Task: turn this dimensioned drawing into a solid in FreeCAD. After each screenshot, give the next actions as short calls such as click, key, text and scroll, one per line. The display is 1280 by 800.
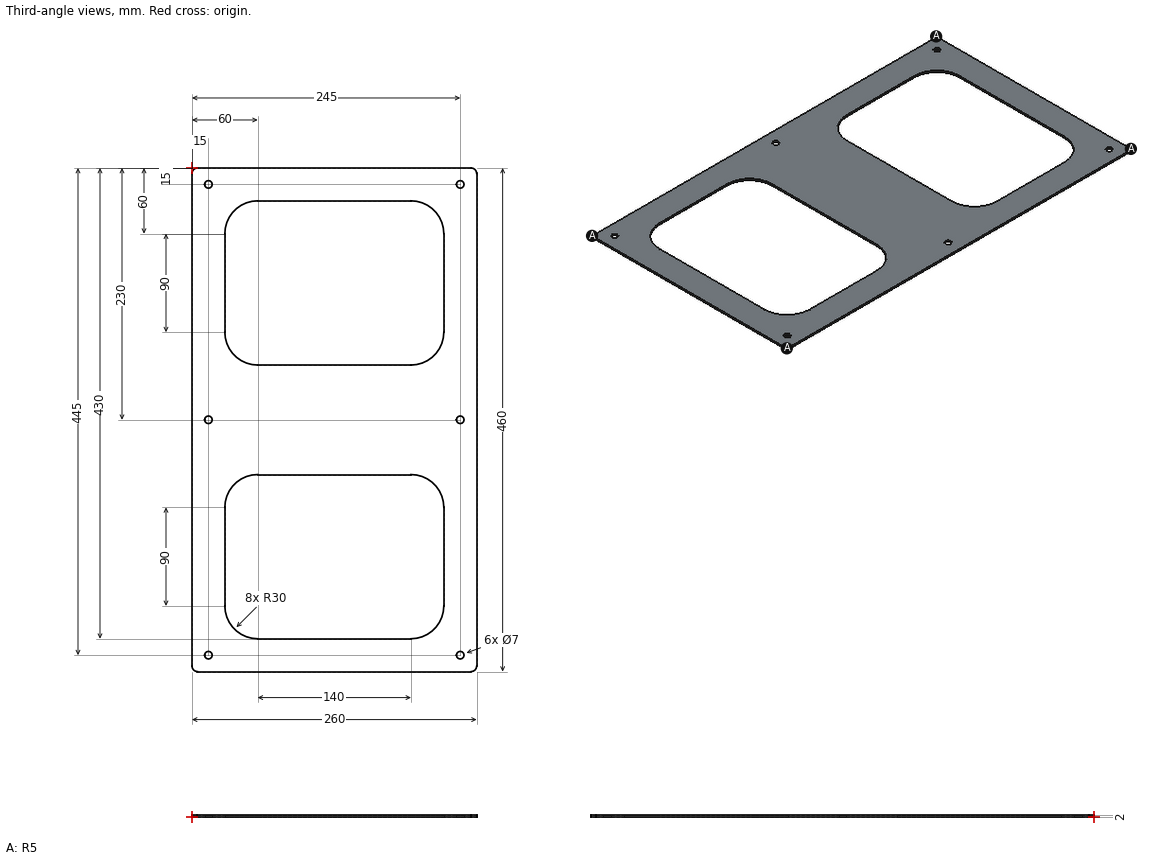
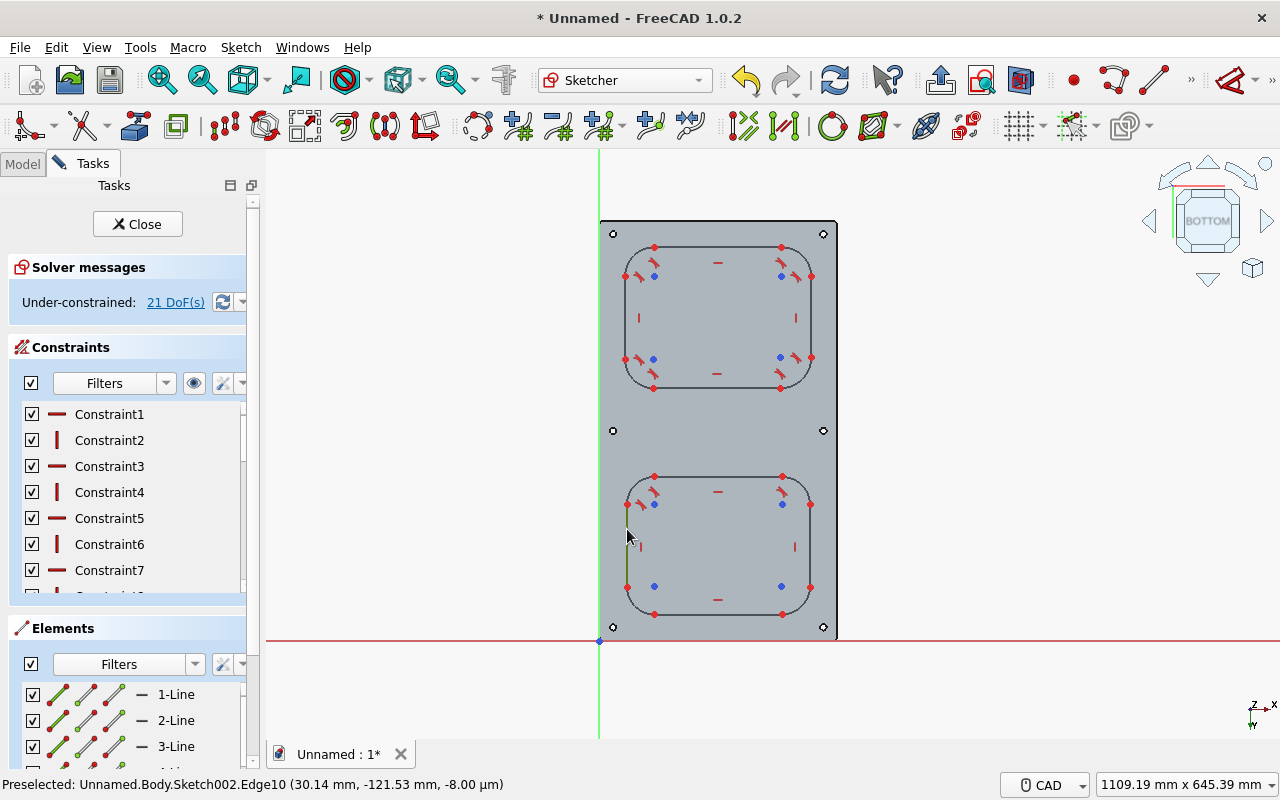
click(630, 600)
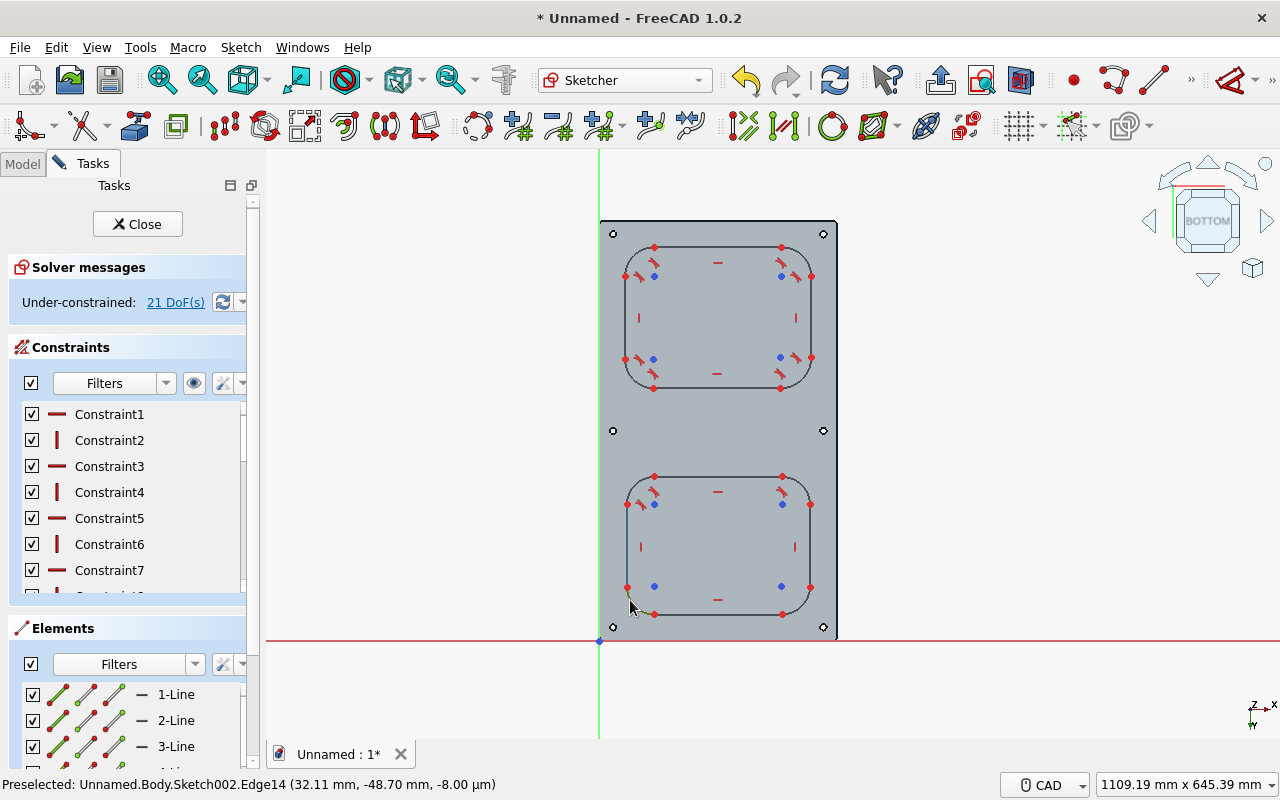
key(t)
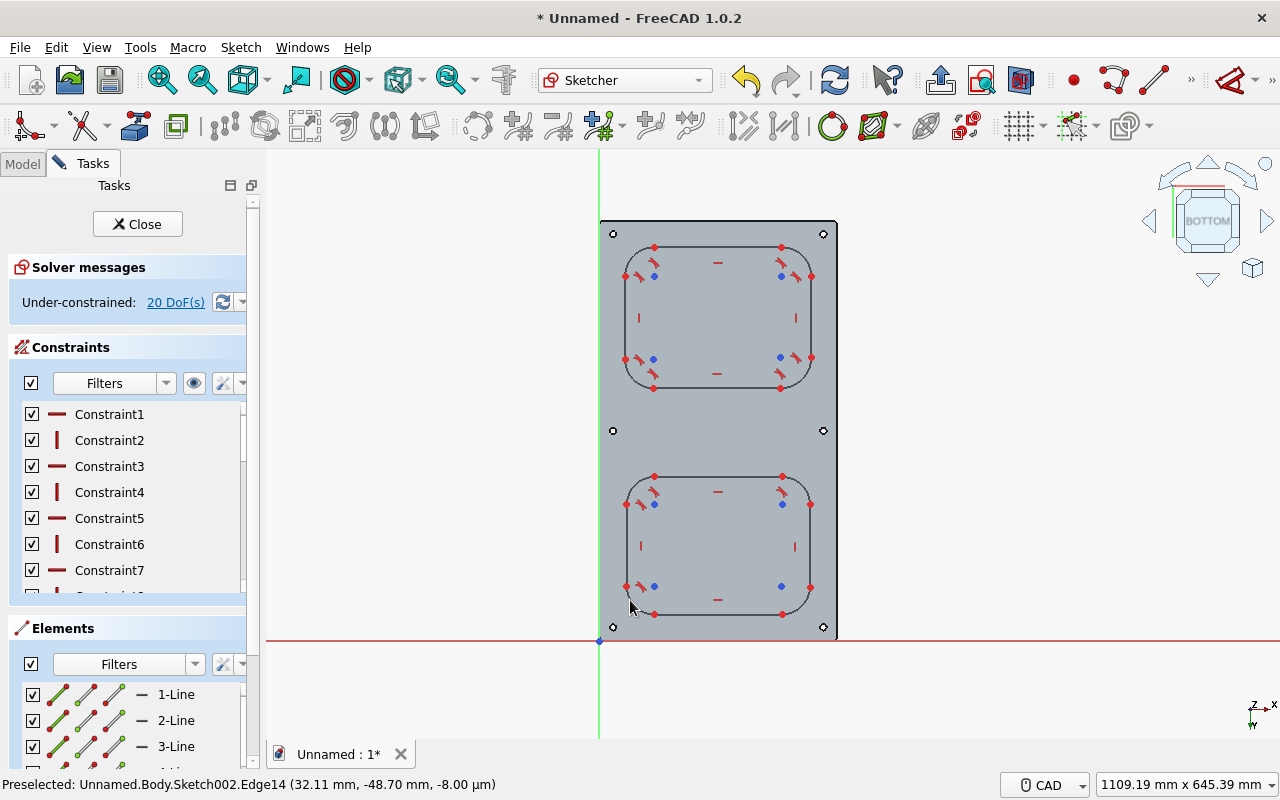
click(692, 615)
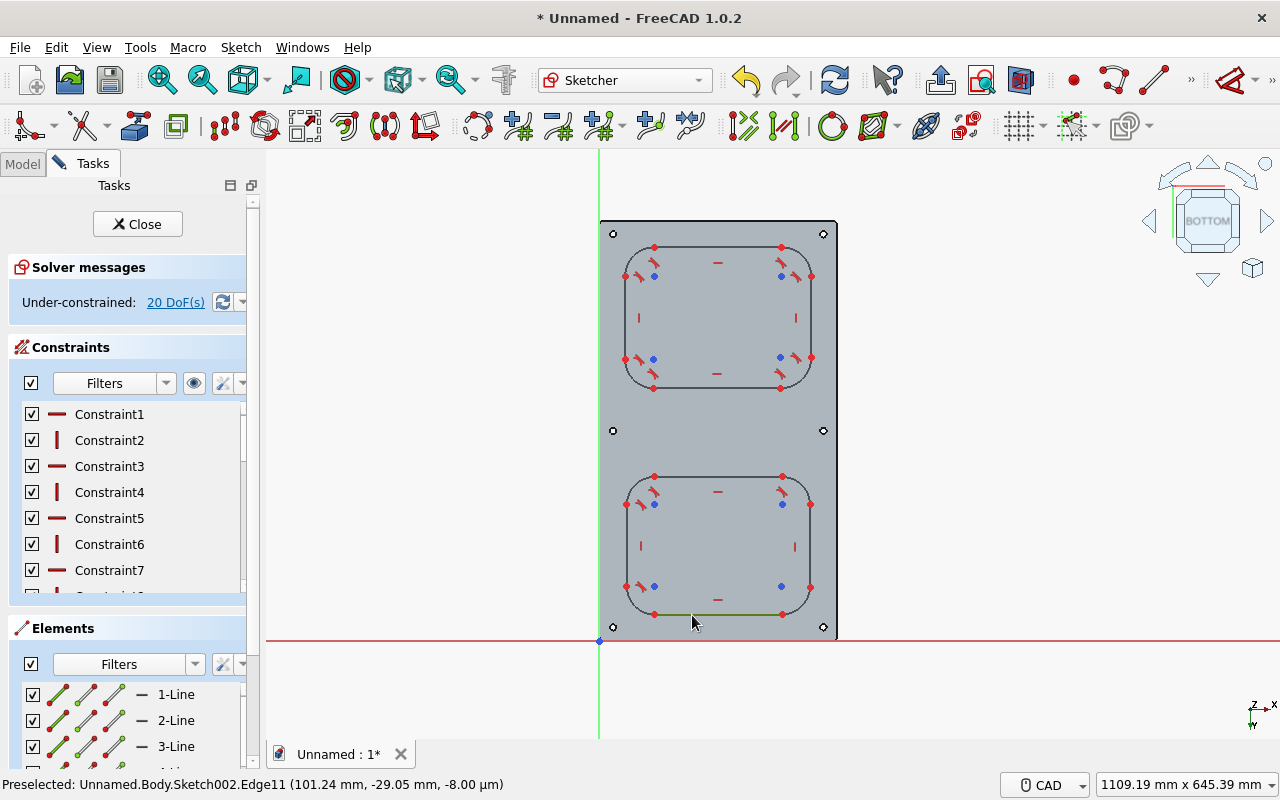
click(630, 599)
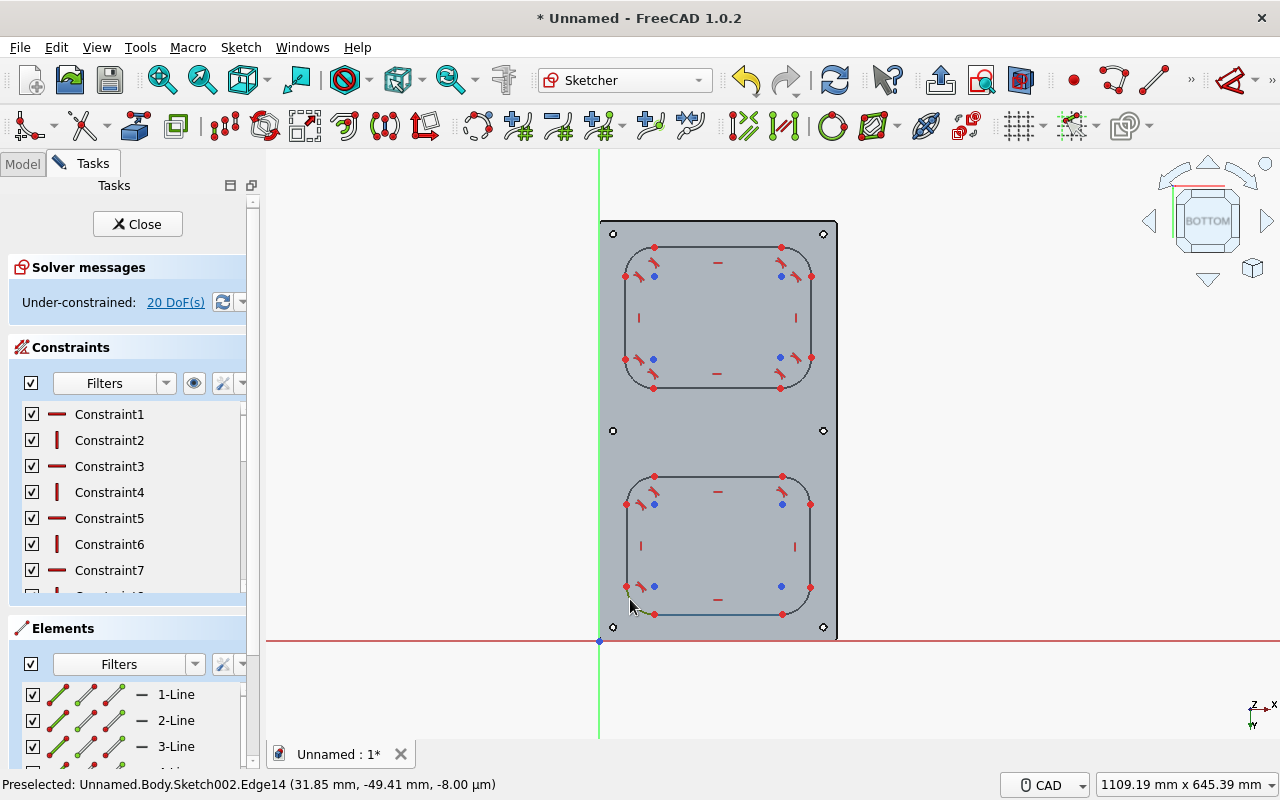
key(t)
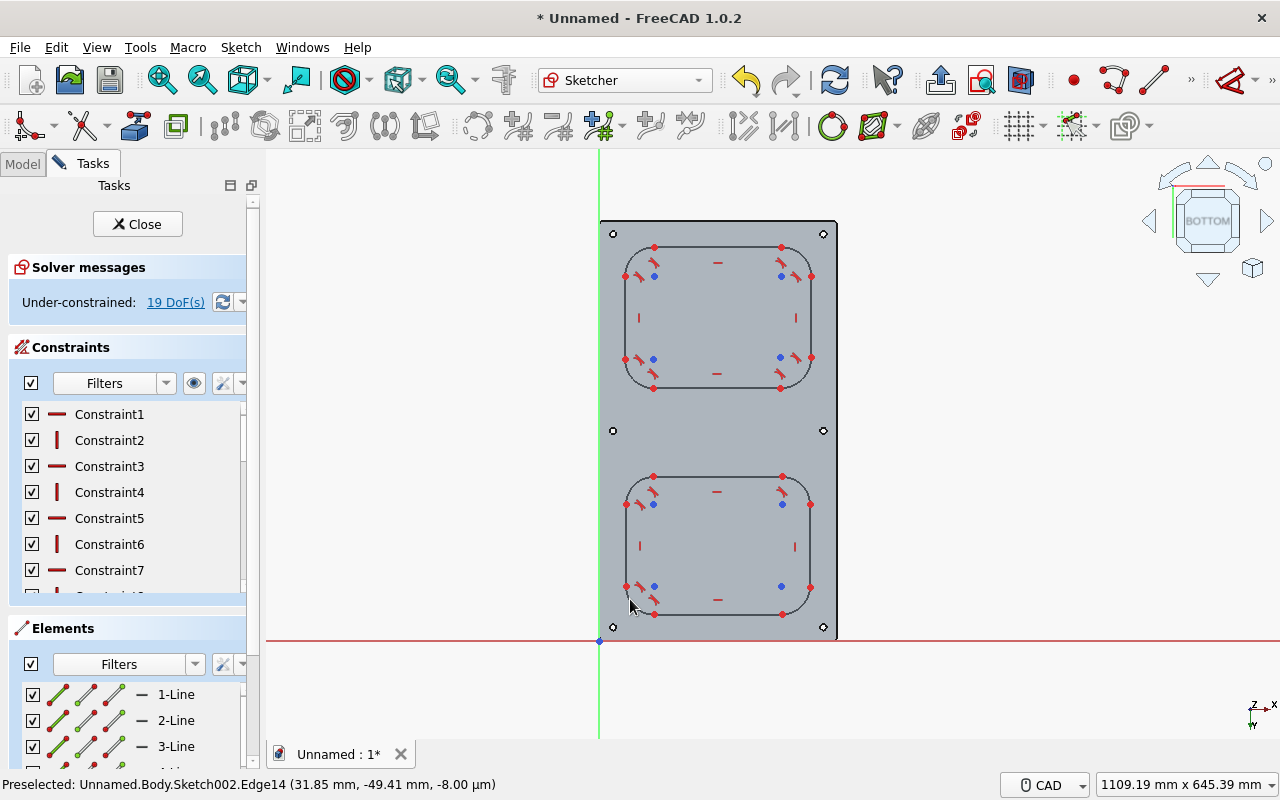
click(692, 615)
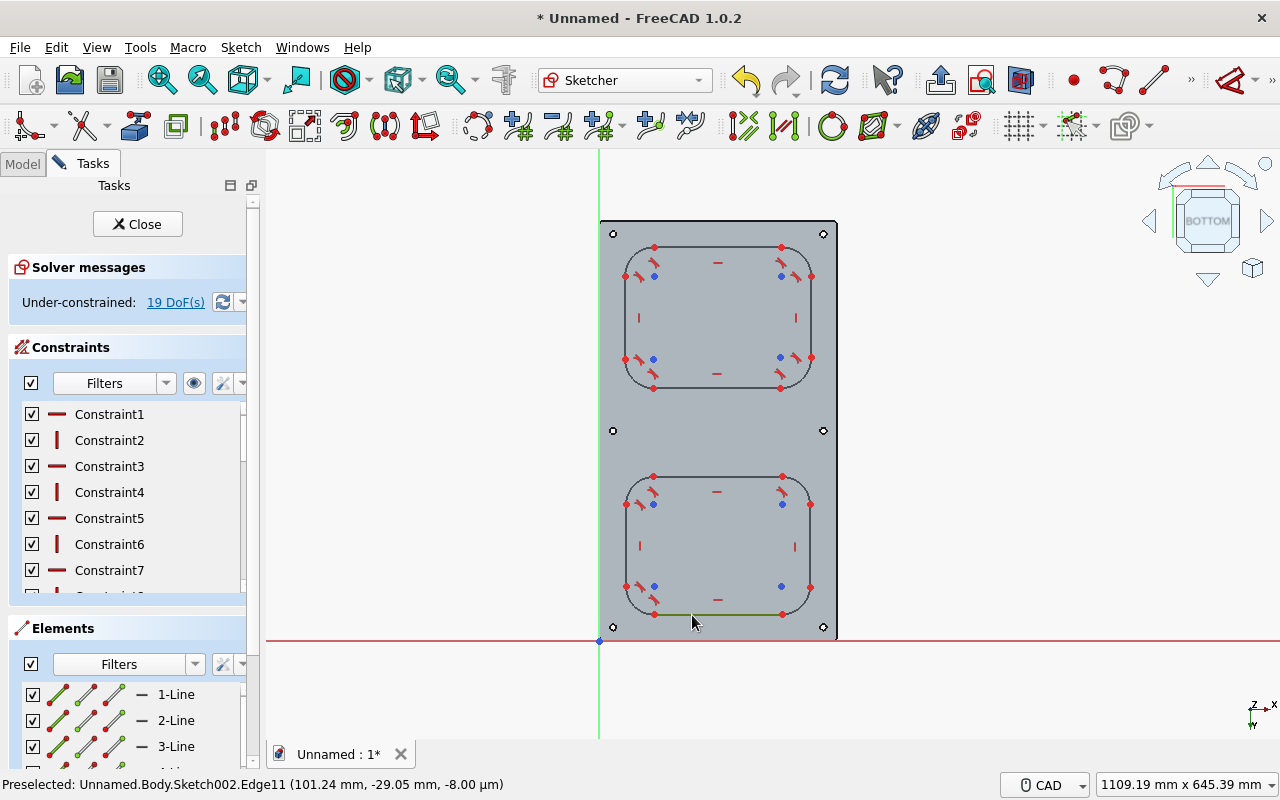
click(794, 611)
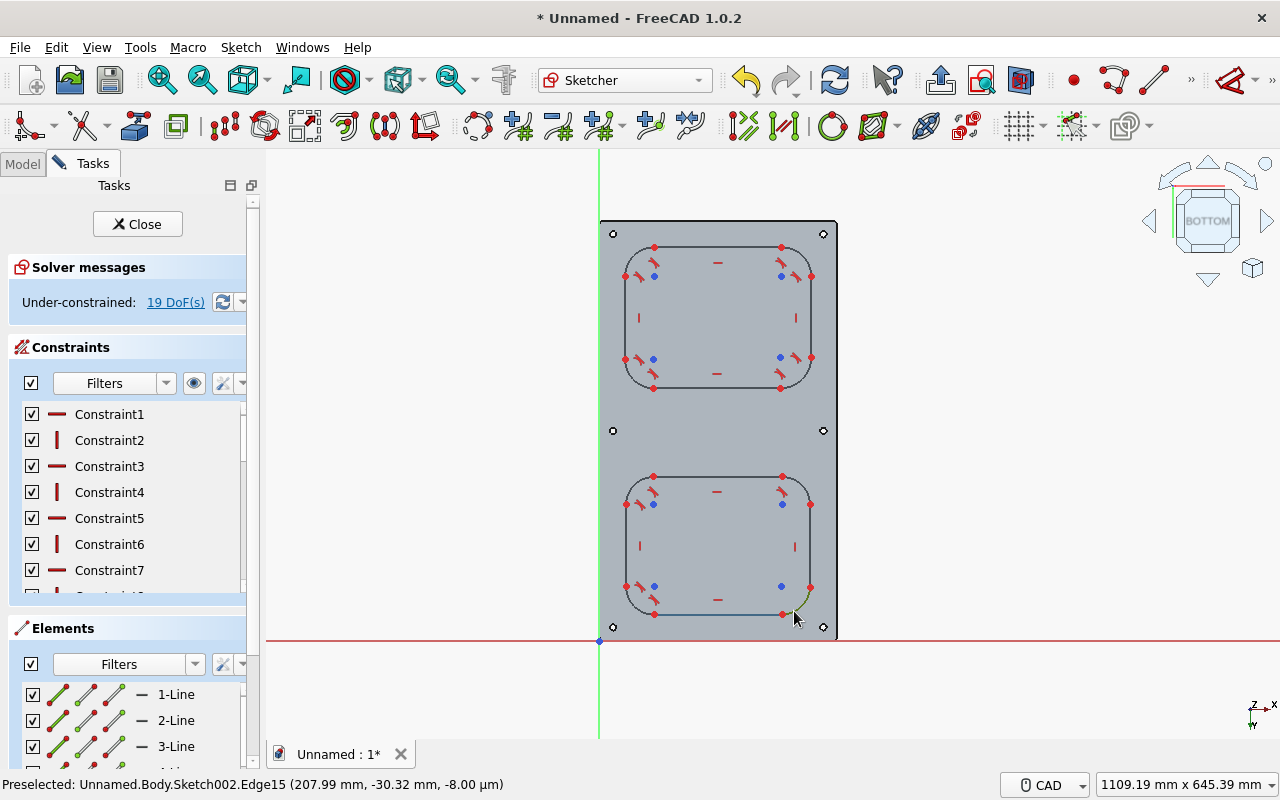
key(t)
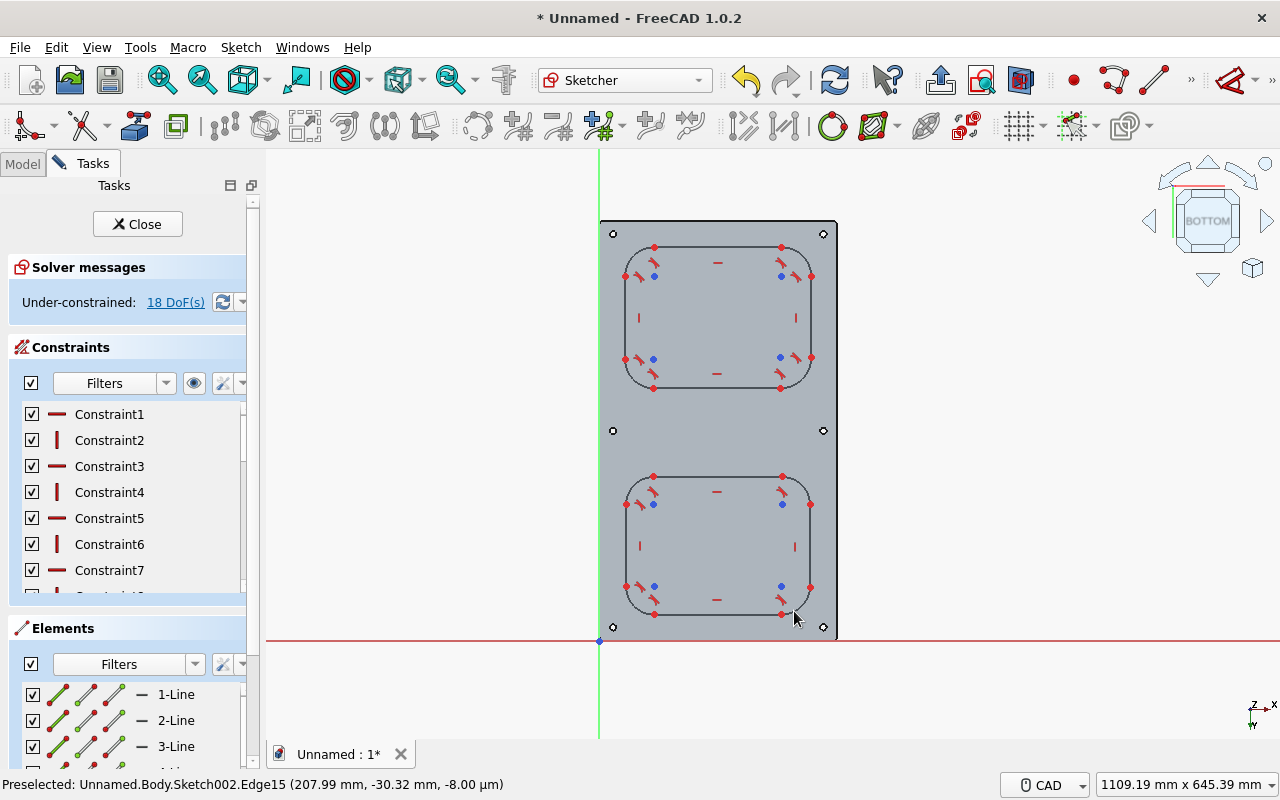
click(810, 563)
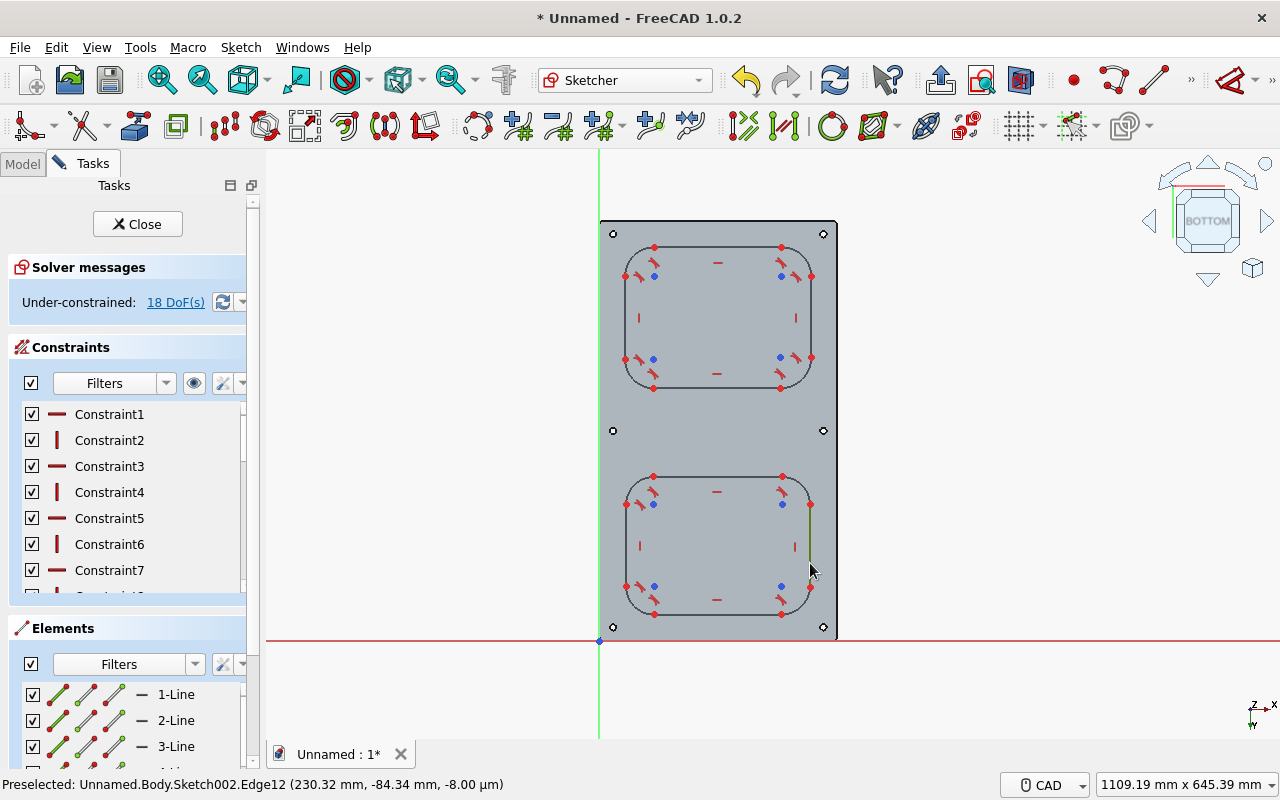
click(794, 612)